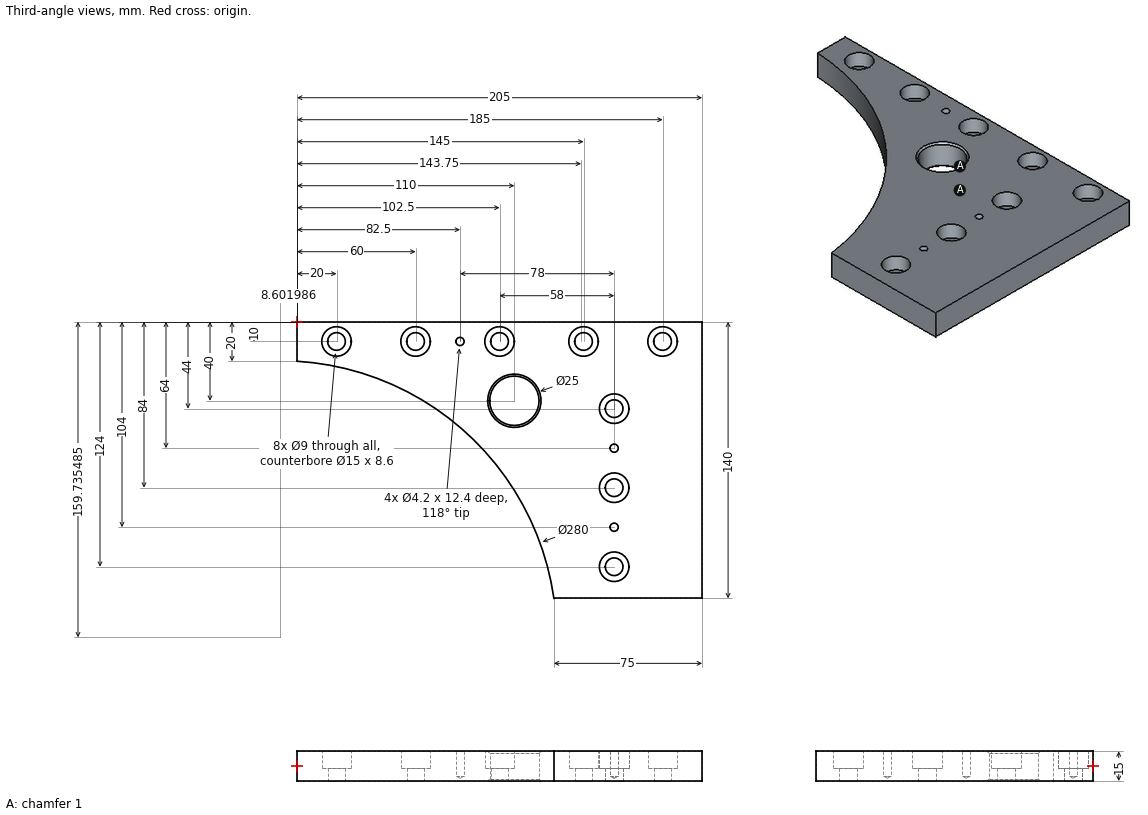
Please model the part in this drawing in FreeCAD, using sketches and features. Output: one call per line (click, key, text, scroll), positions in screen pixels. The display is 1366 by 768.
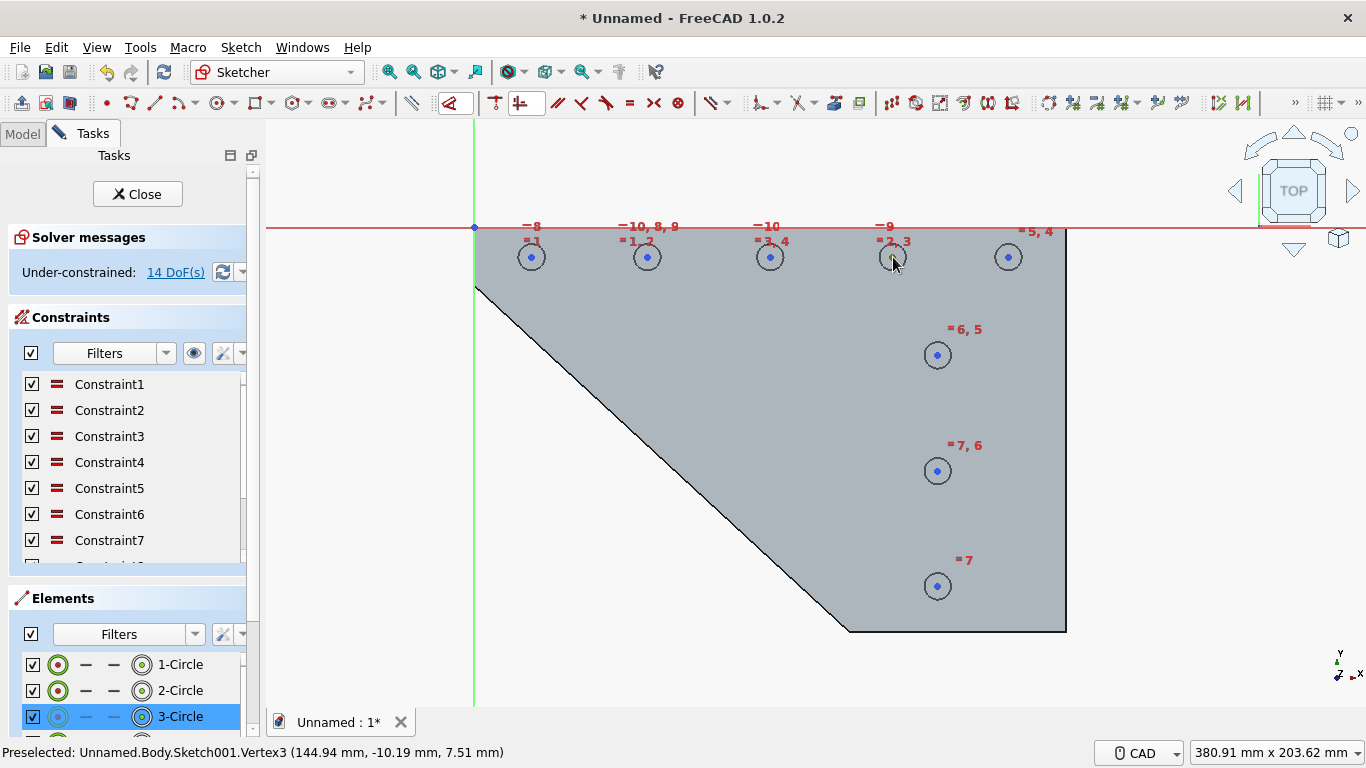
click(1009, 257)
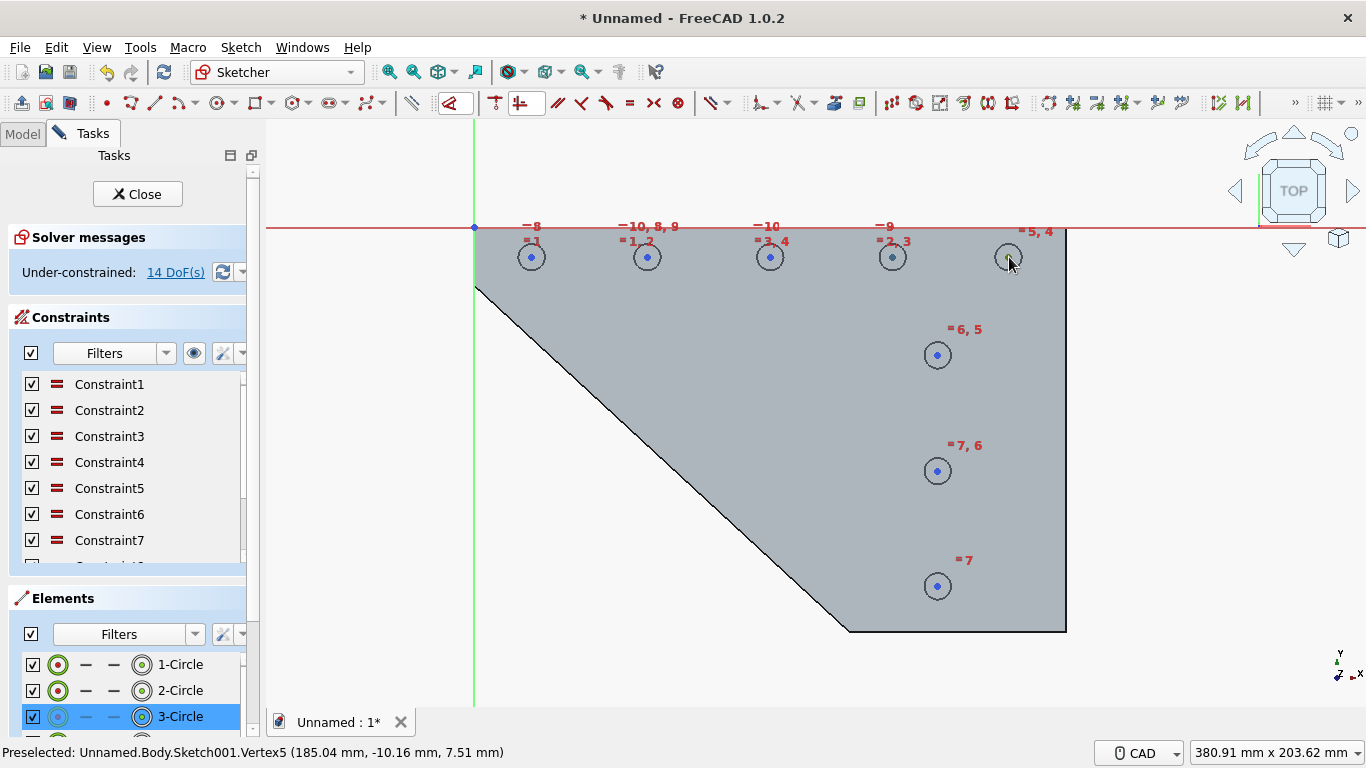
key(h)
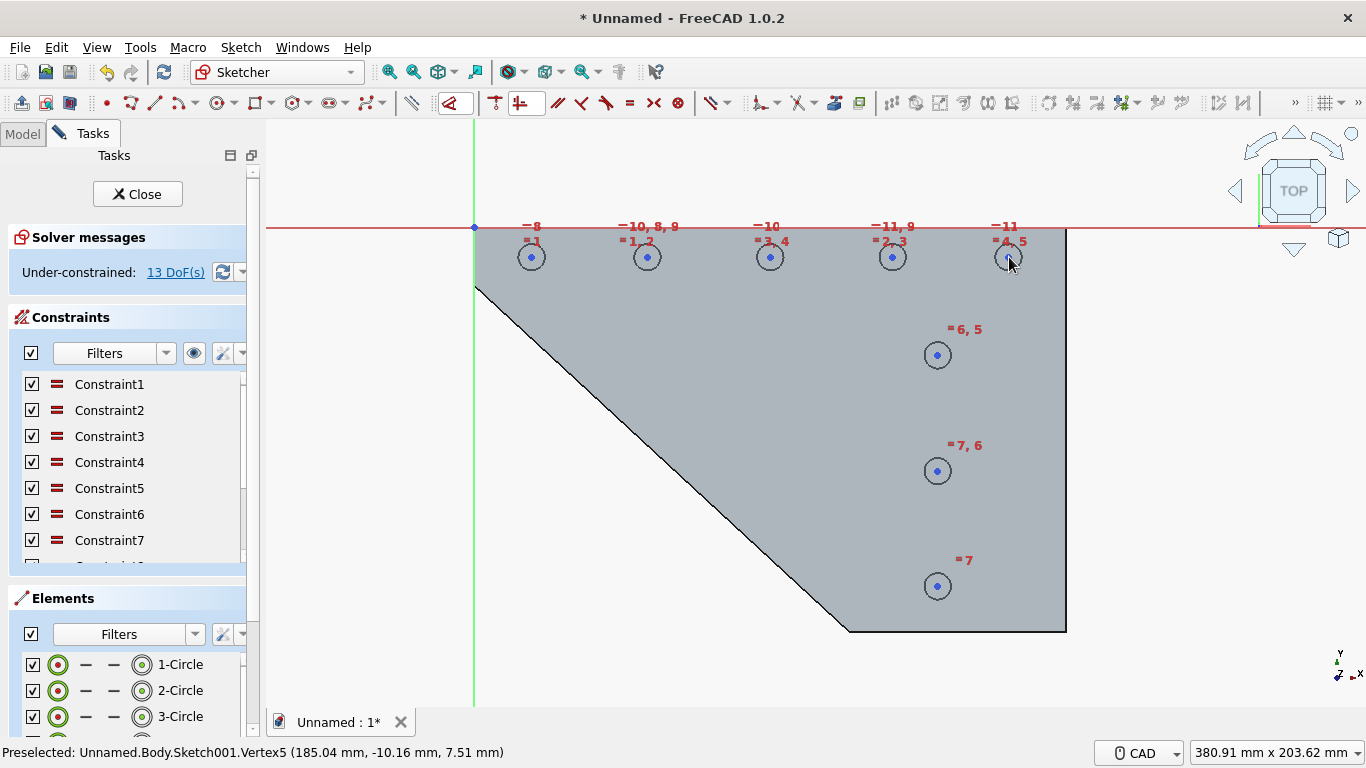
click(938, 355)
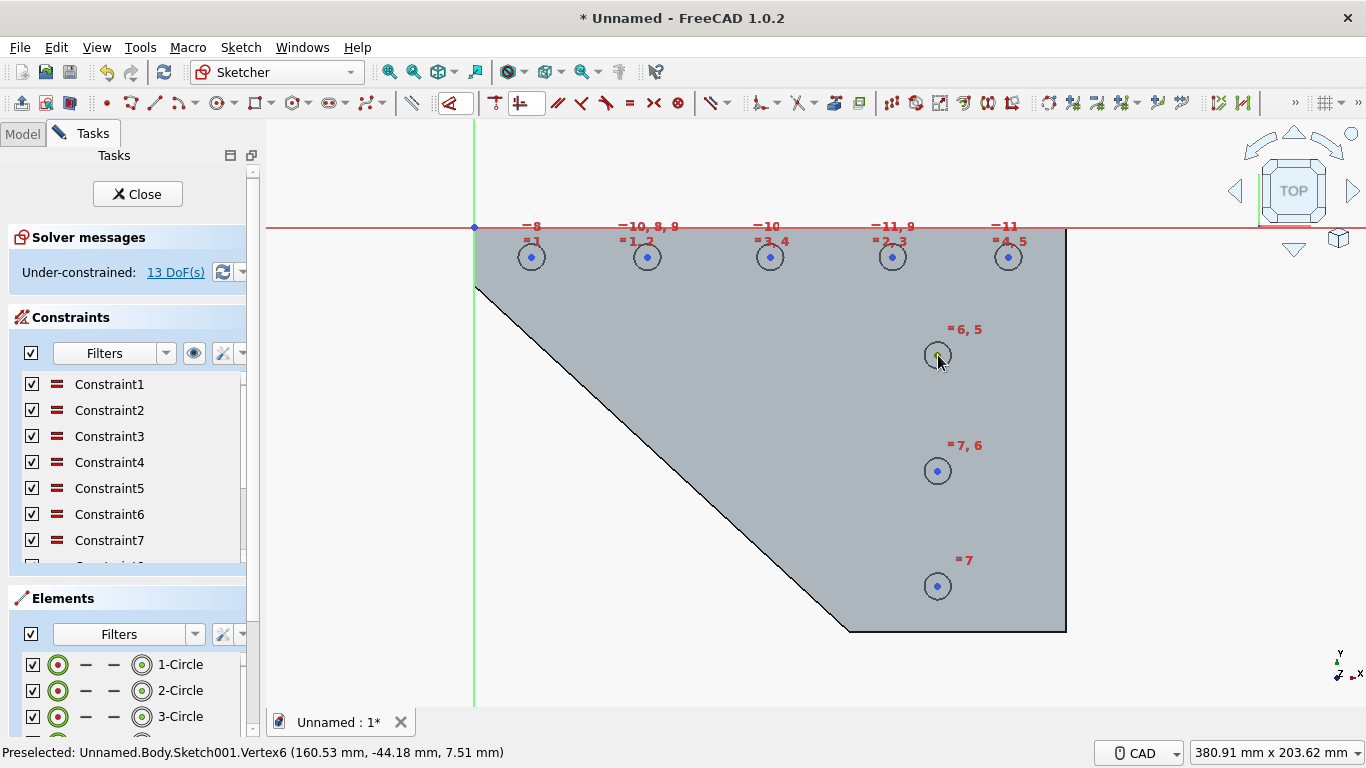
click(938, 471)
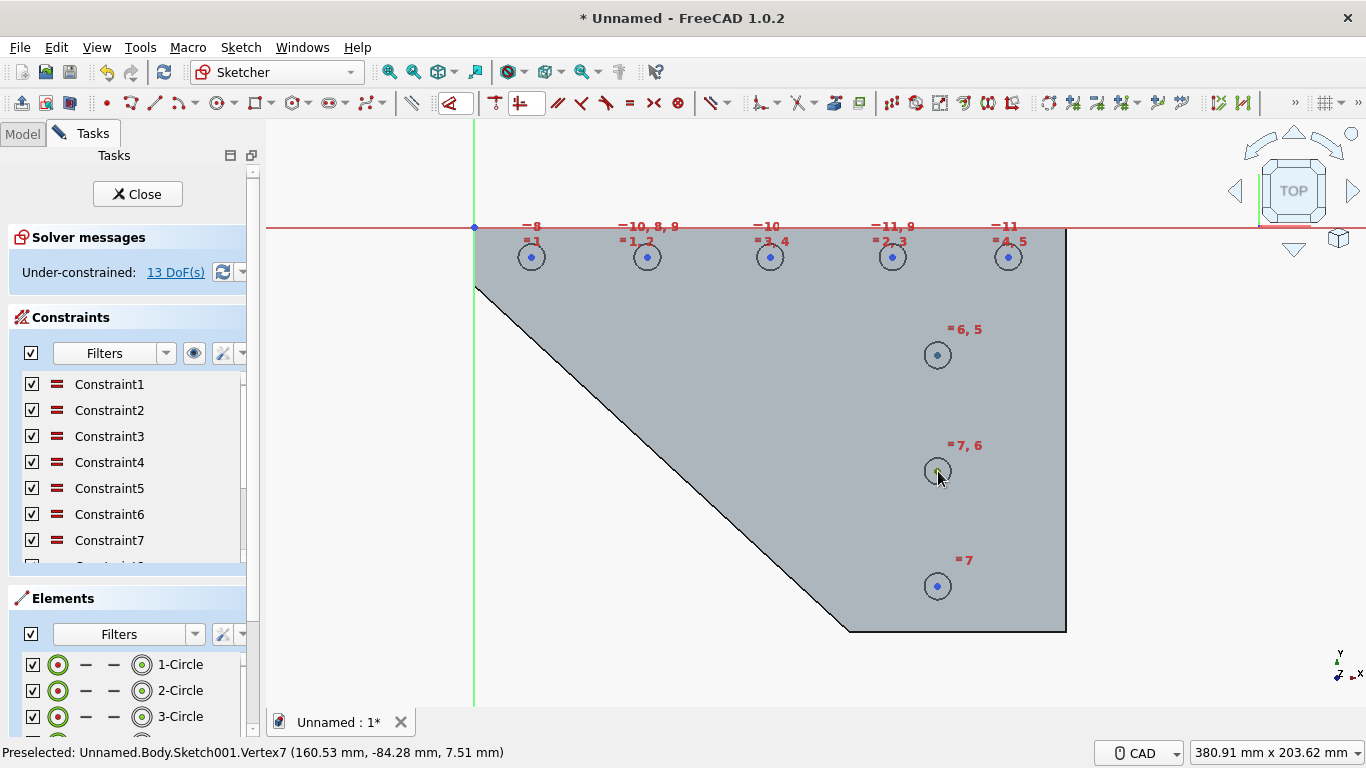
key(v)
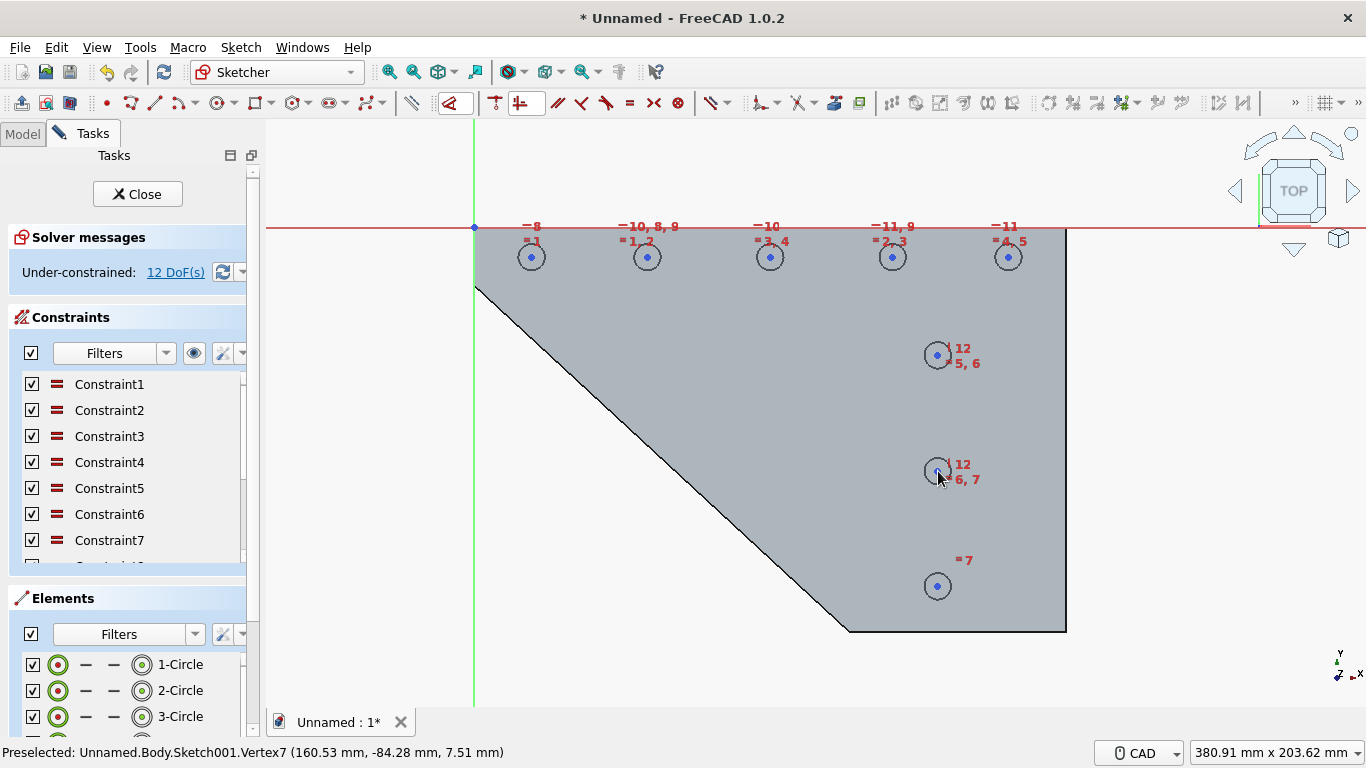
click(938, 471)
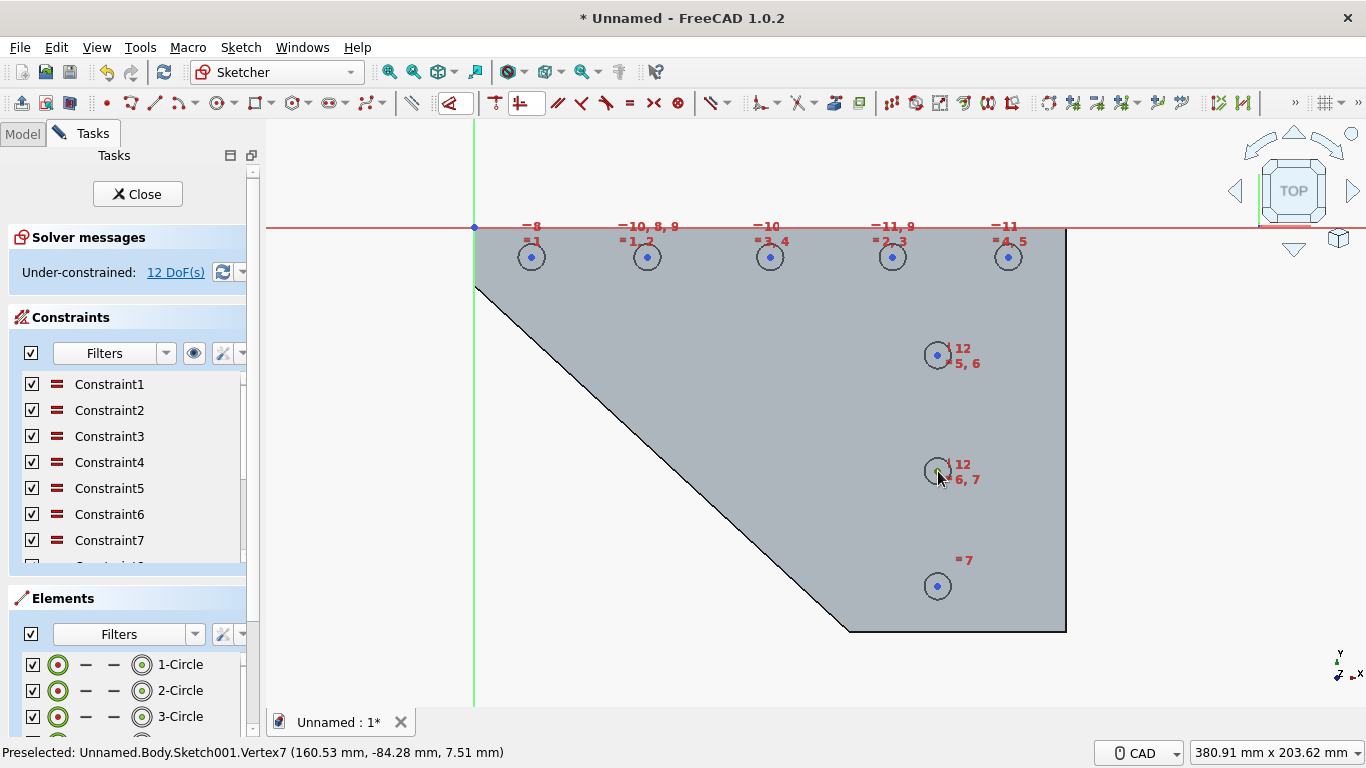
click(938, 586)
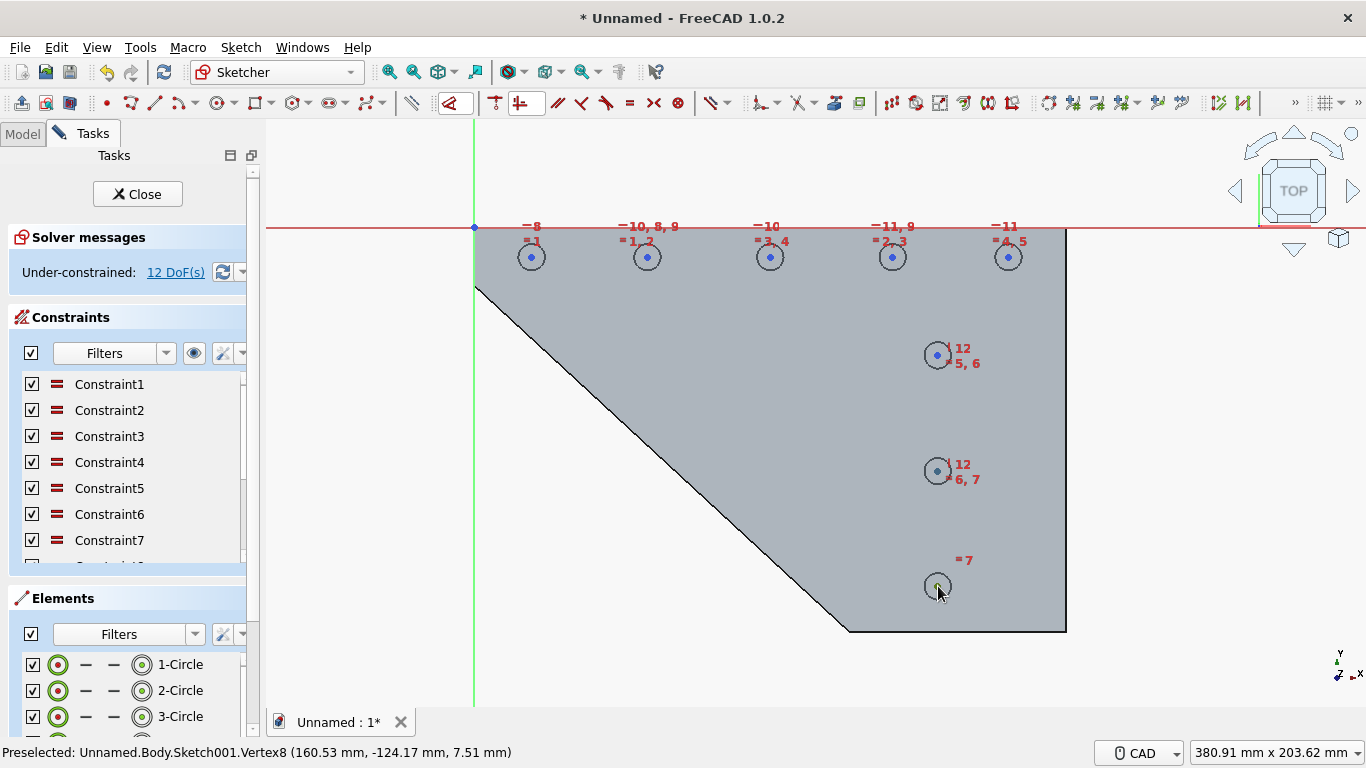
click(540, 104)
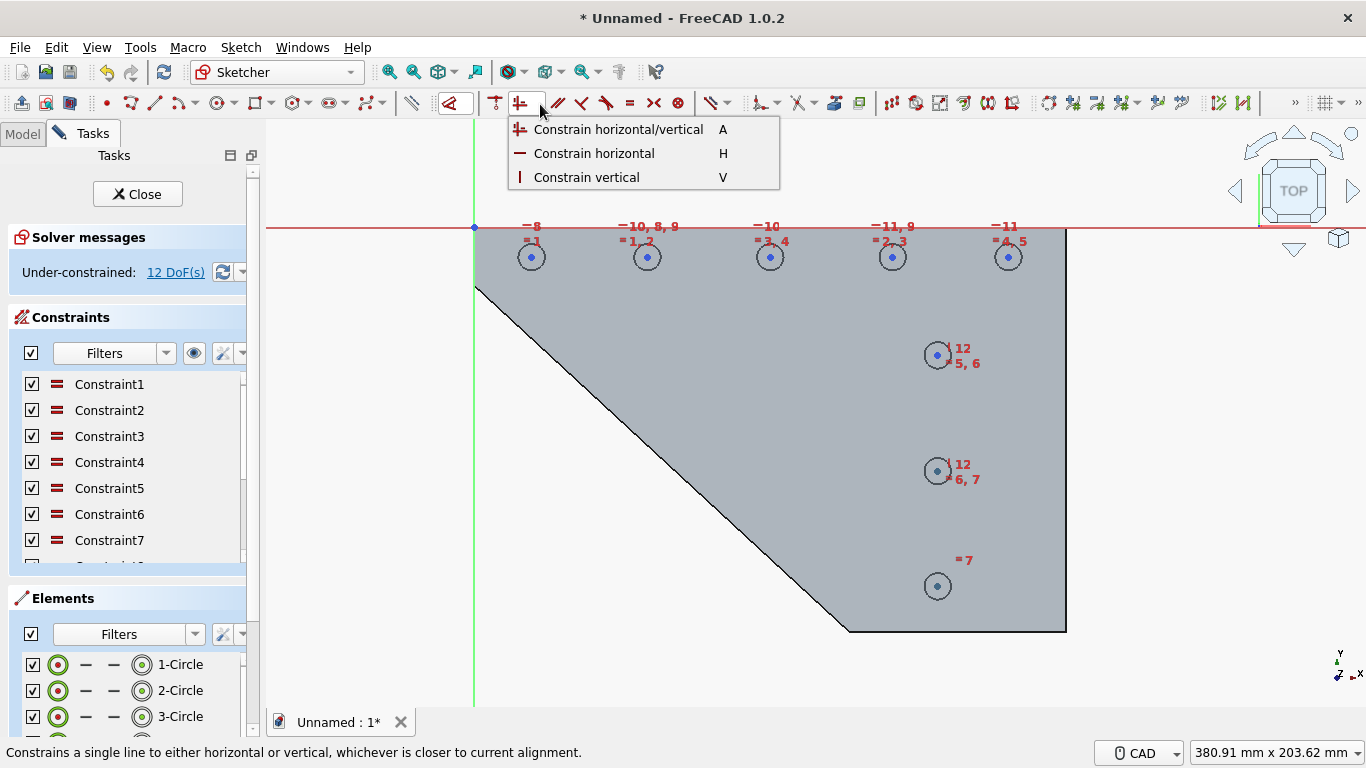
click(644, 177)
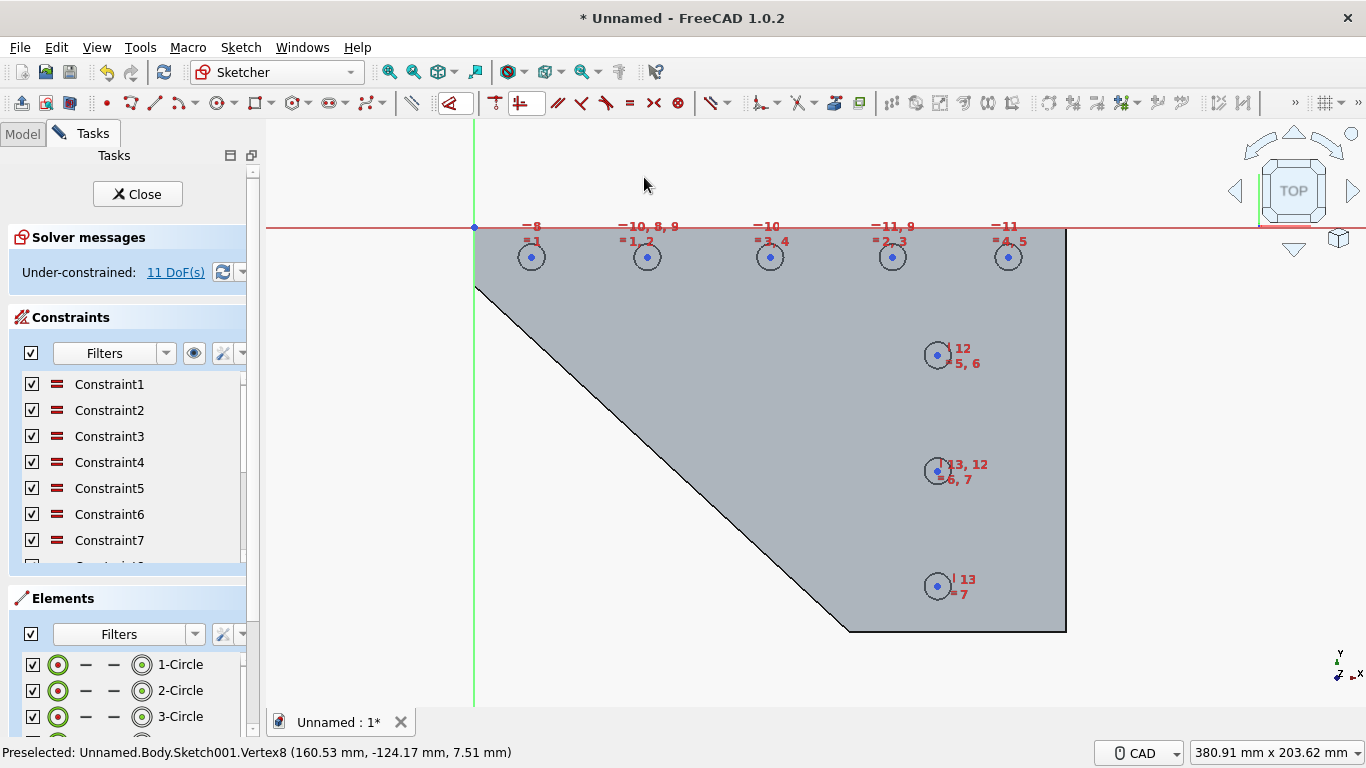
scroll(541, 248, up, 3)